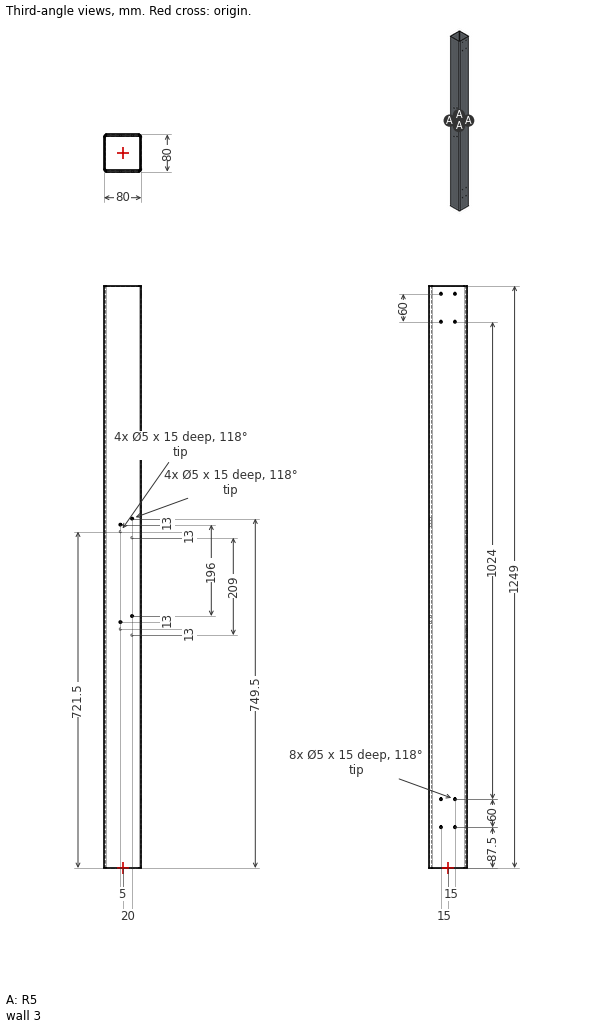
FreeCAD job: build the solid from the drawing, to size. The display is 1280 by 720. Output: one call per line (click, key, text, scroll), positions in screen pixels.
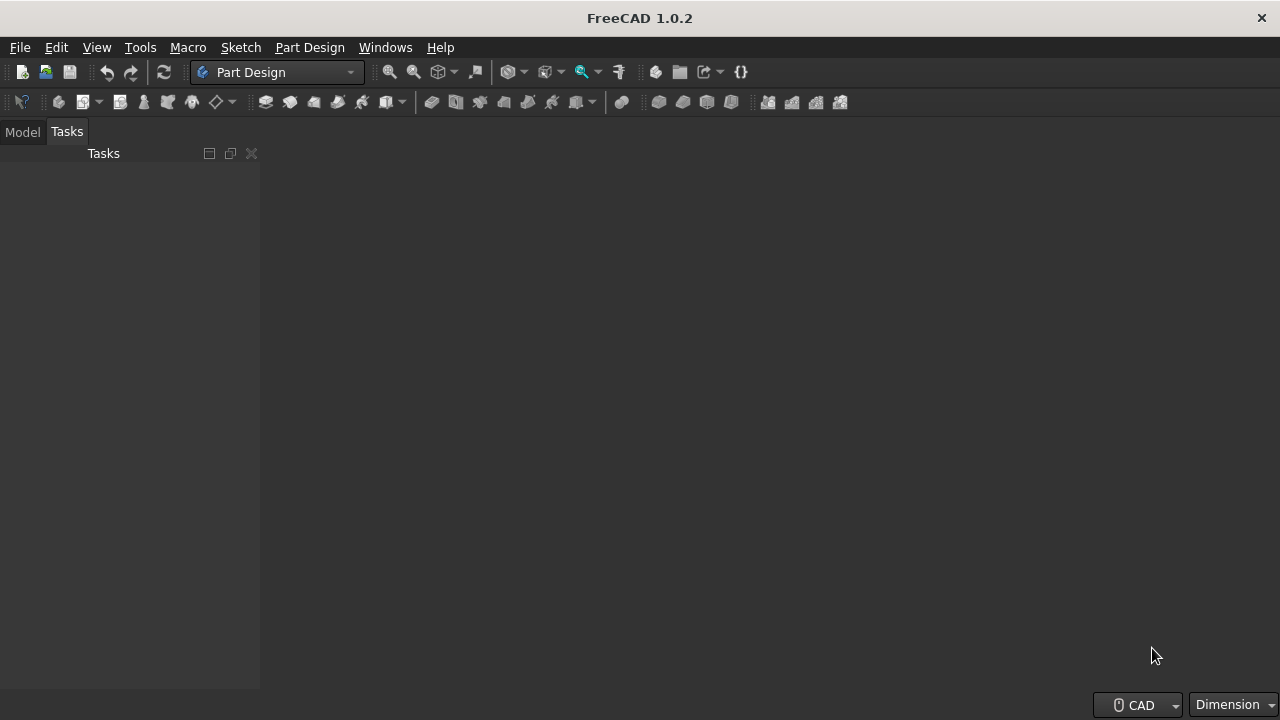
key(ctrl+n)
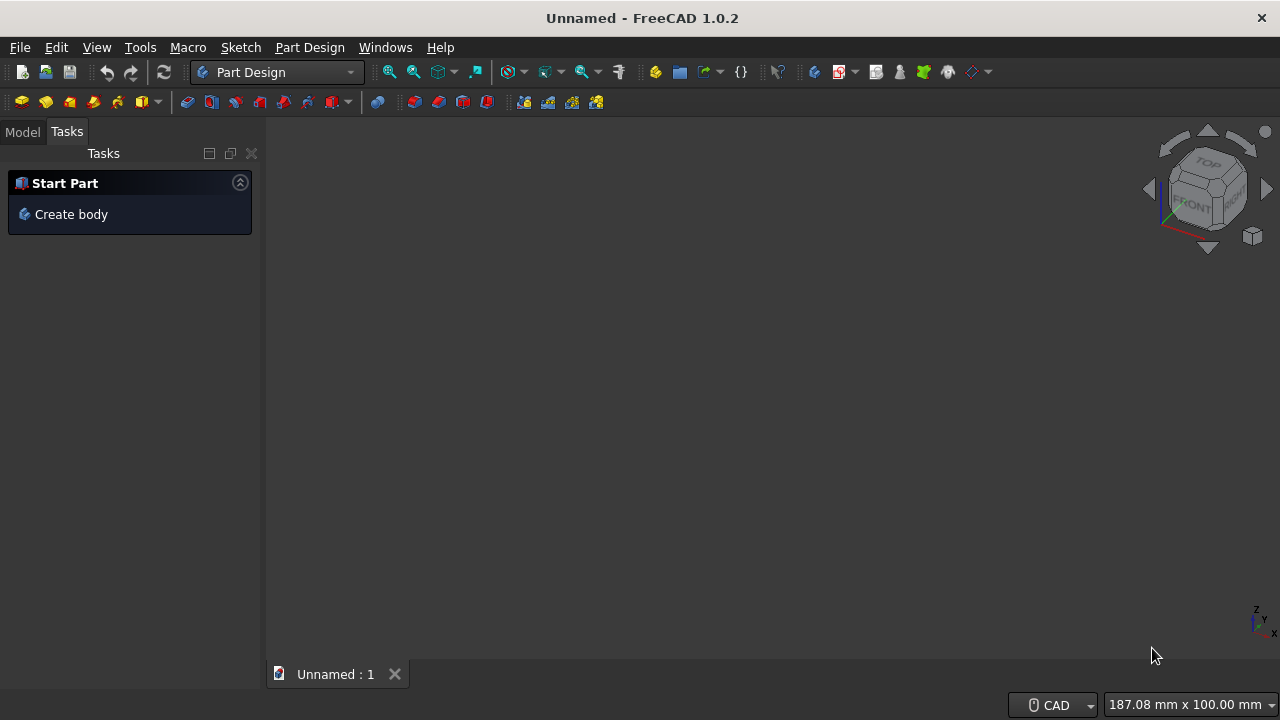
click(840, 72)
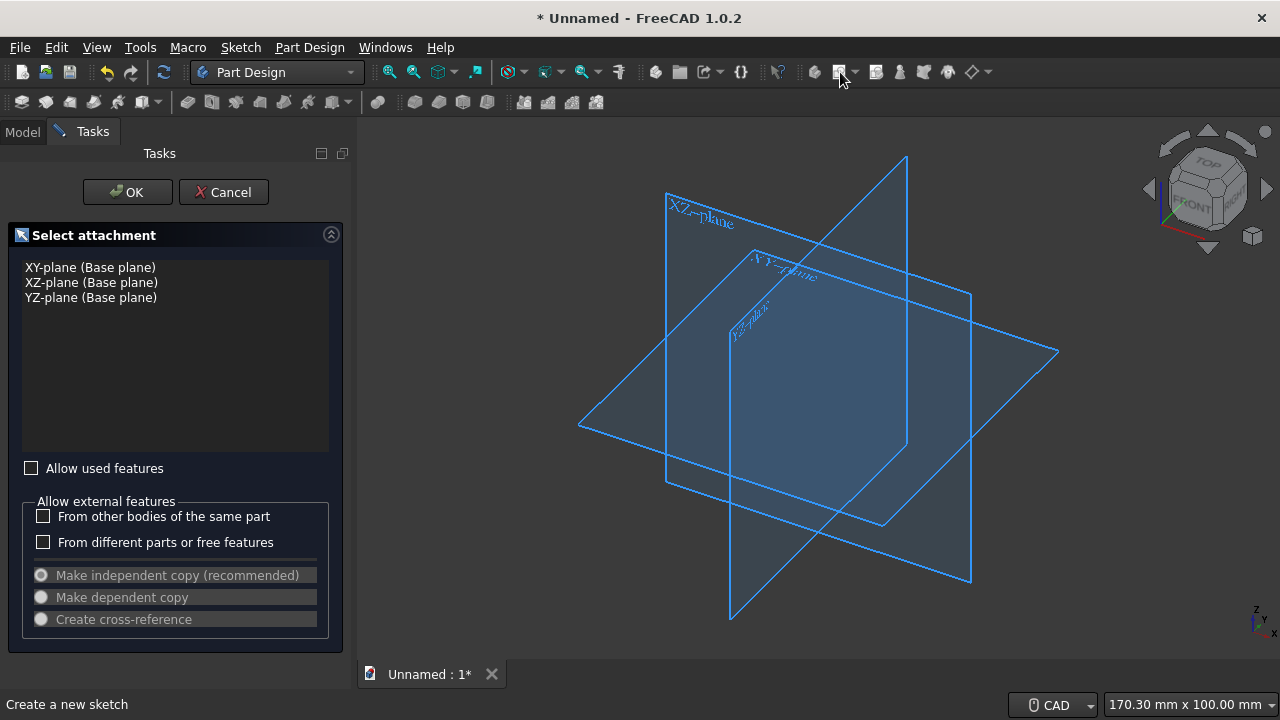
click(82, 268)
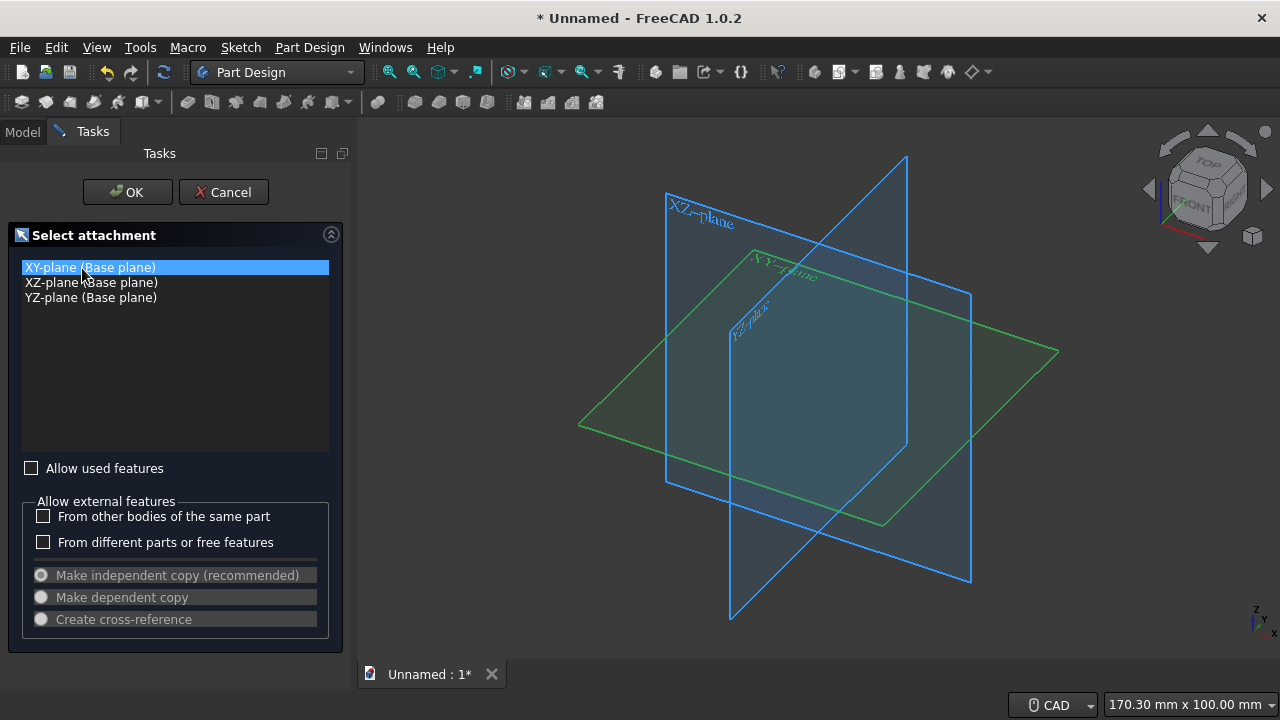
click(128, 192)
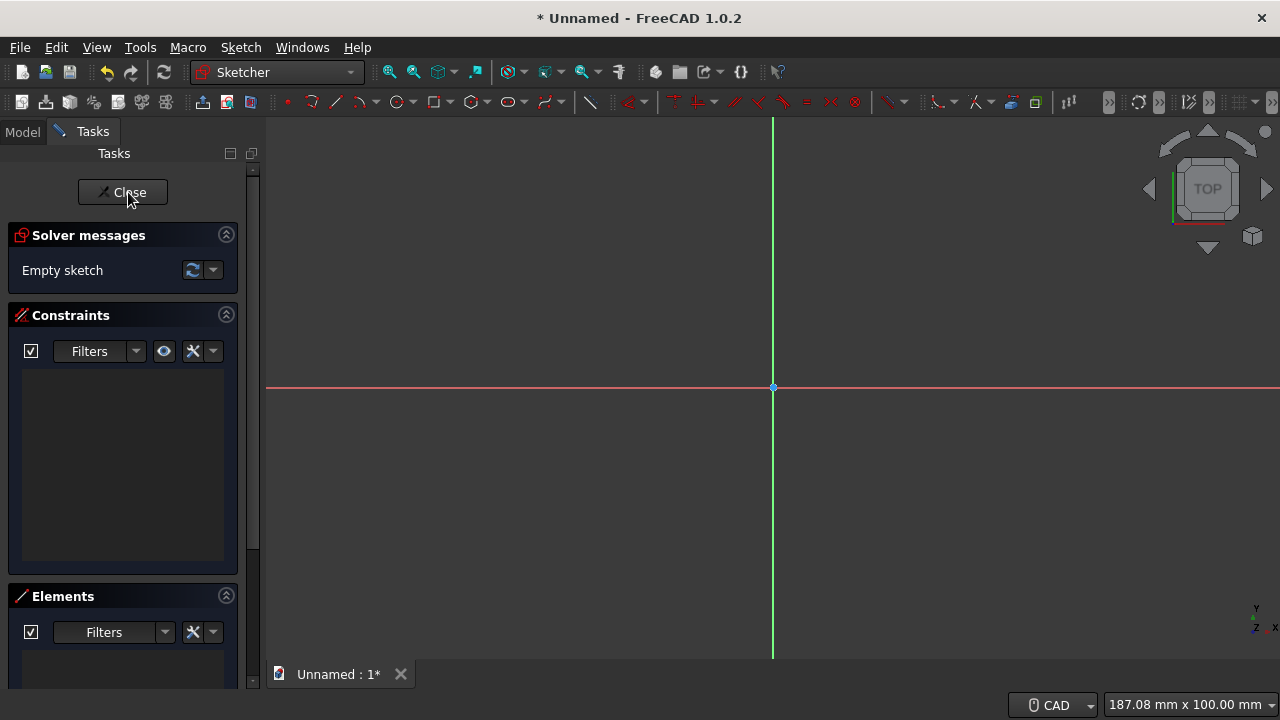
key(g)
key(v)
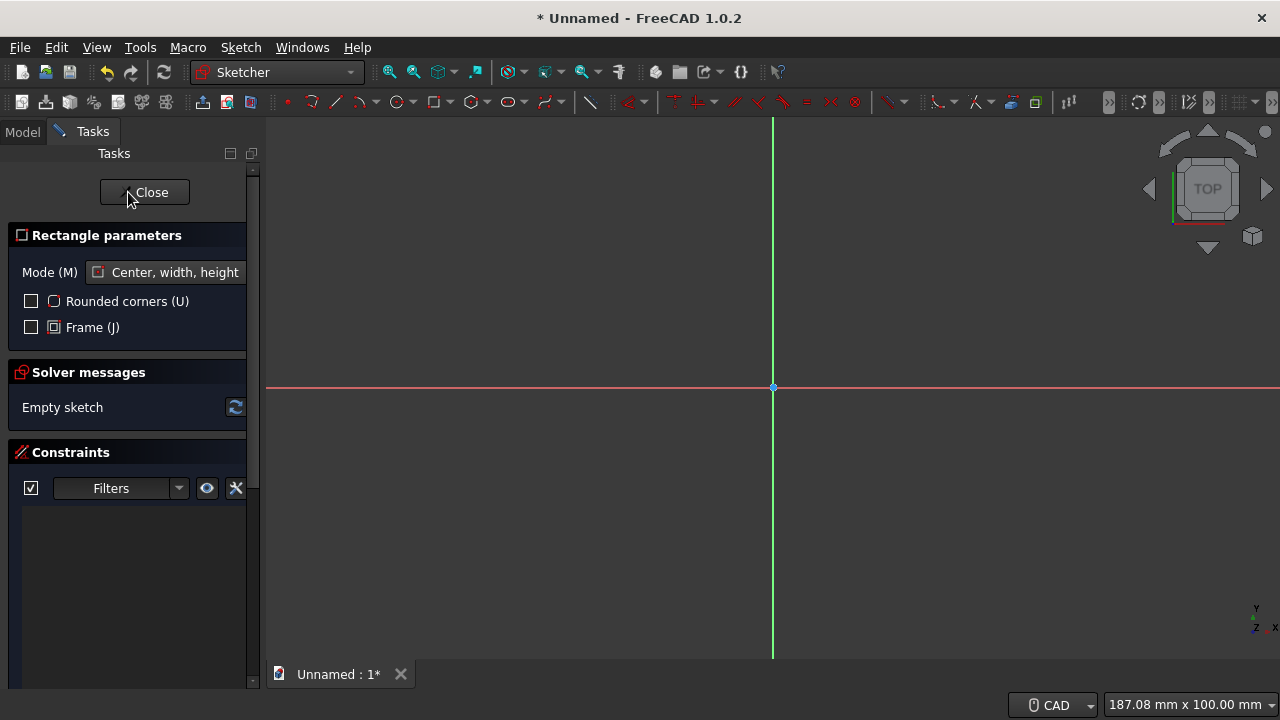
click(773, 388)
move(990, 171)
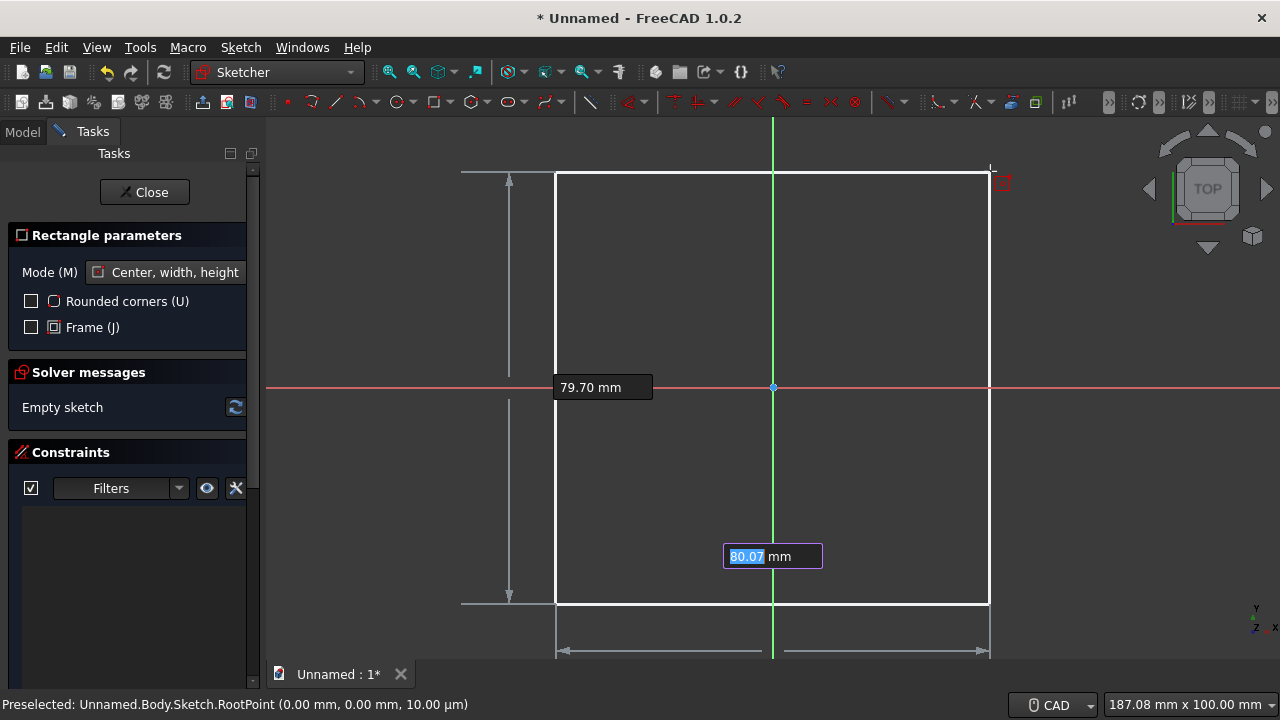
text(80)
key(Tab)
text(80)
key(Return)
key(Escape)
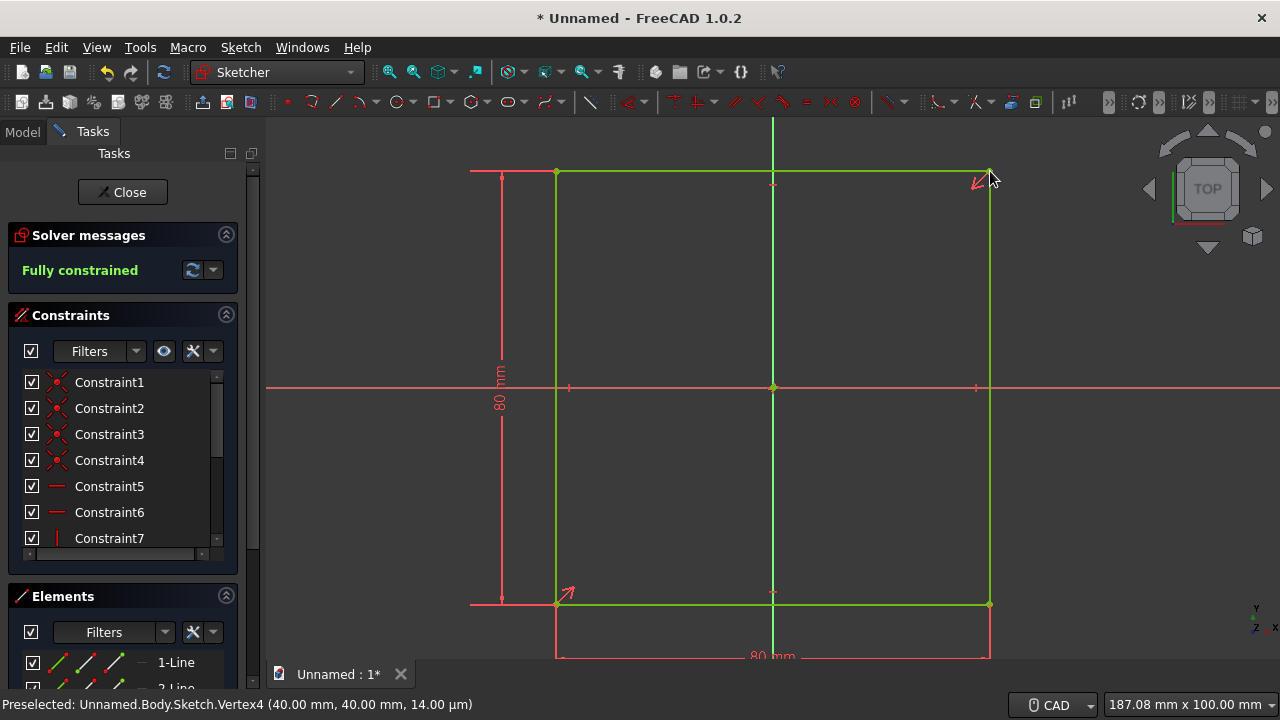
click(123, 192)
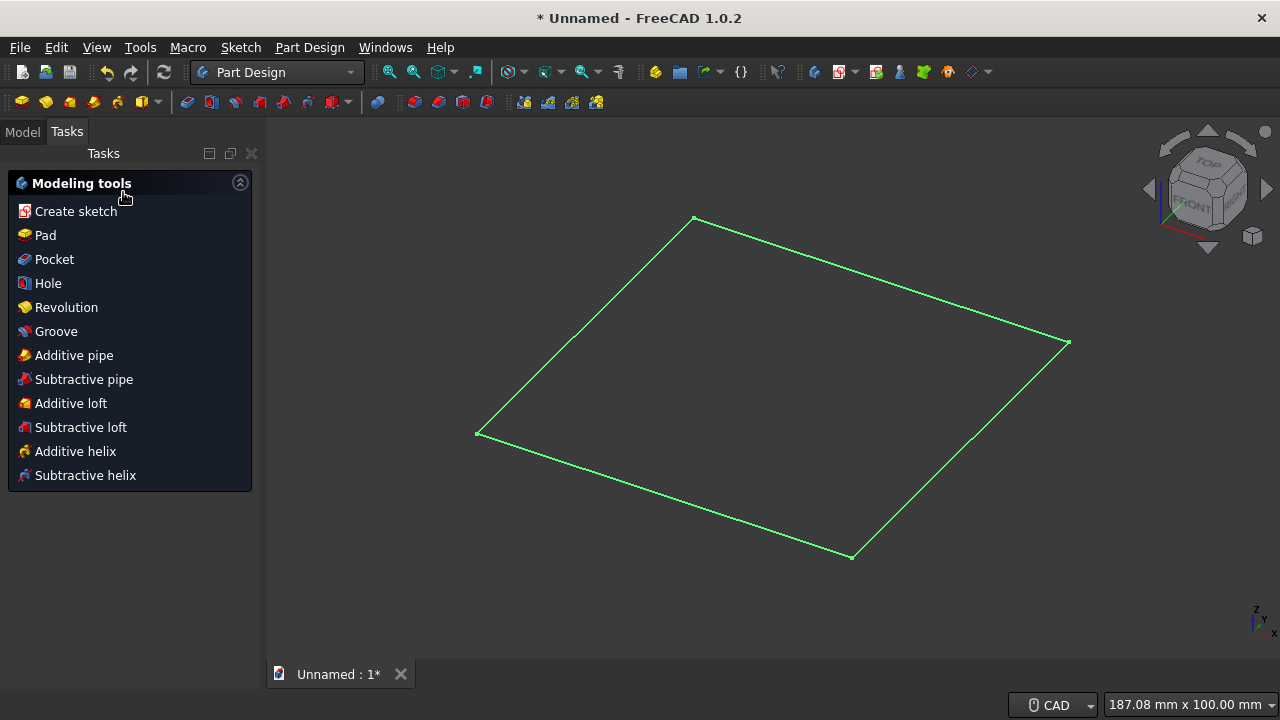
click(22, 102)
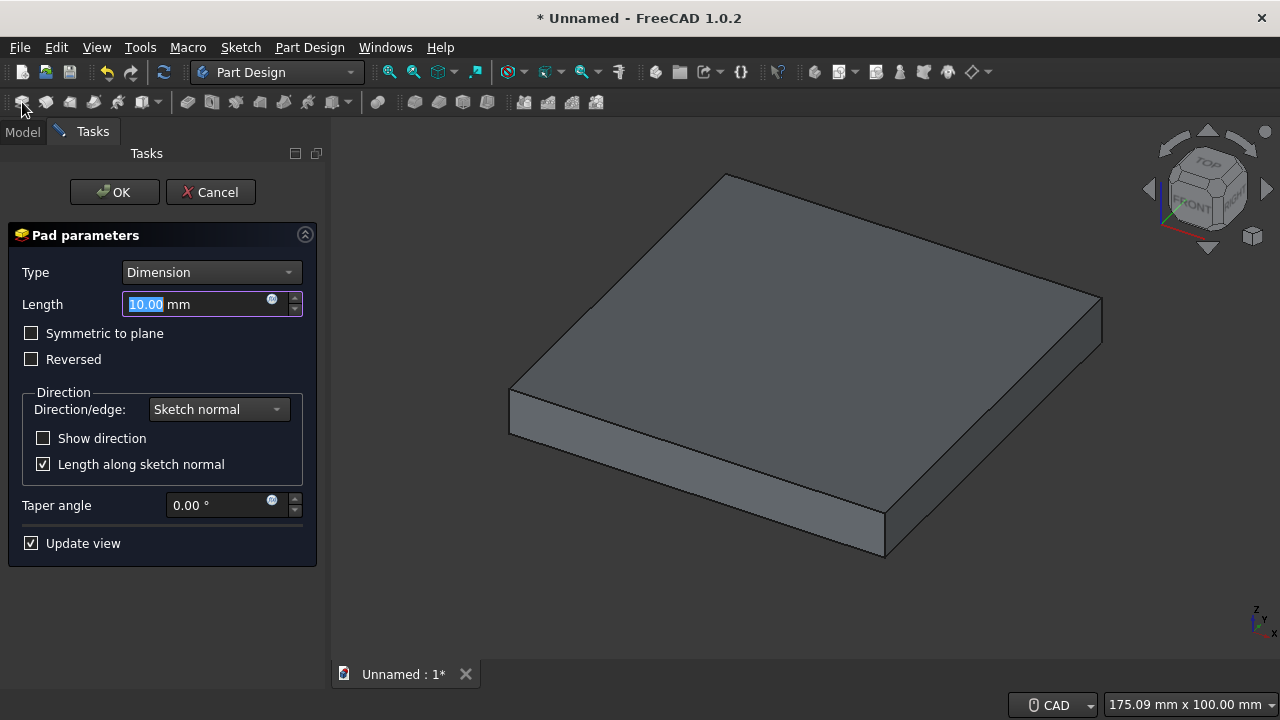
text(1249)
key(Tab)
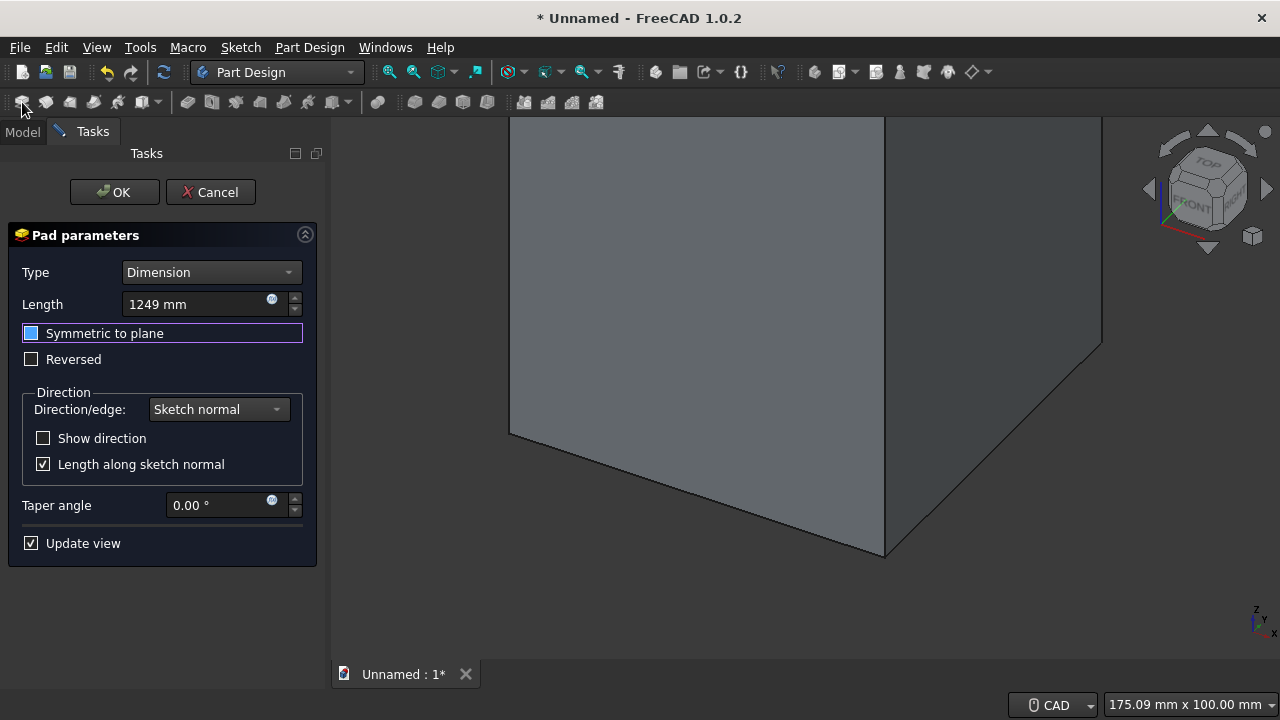
click(115, 192)